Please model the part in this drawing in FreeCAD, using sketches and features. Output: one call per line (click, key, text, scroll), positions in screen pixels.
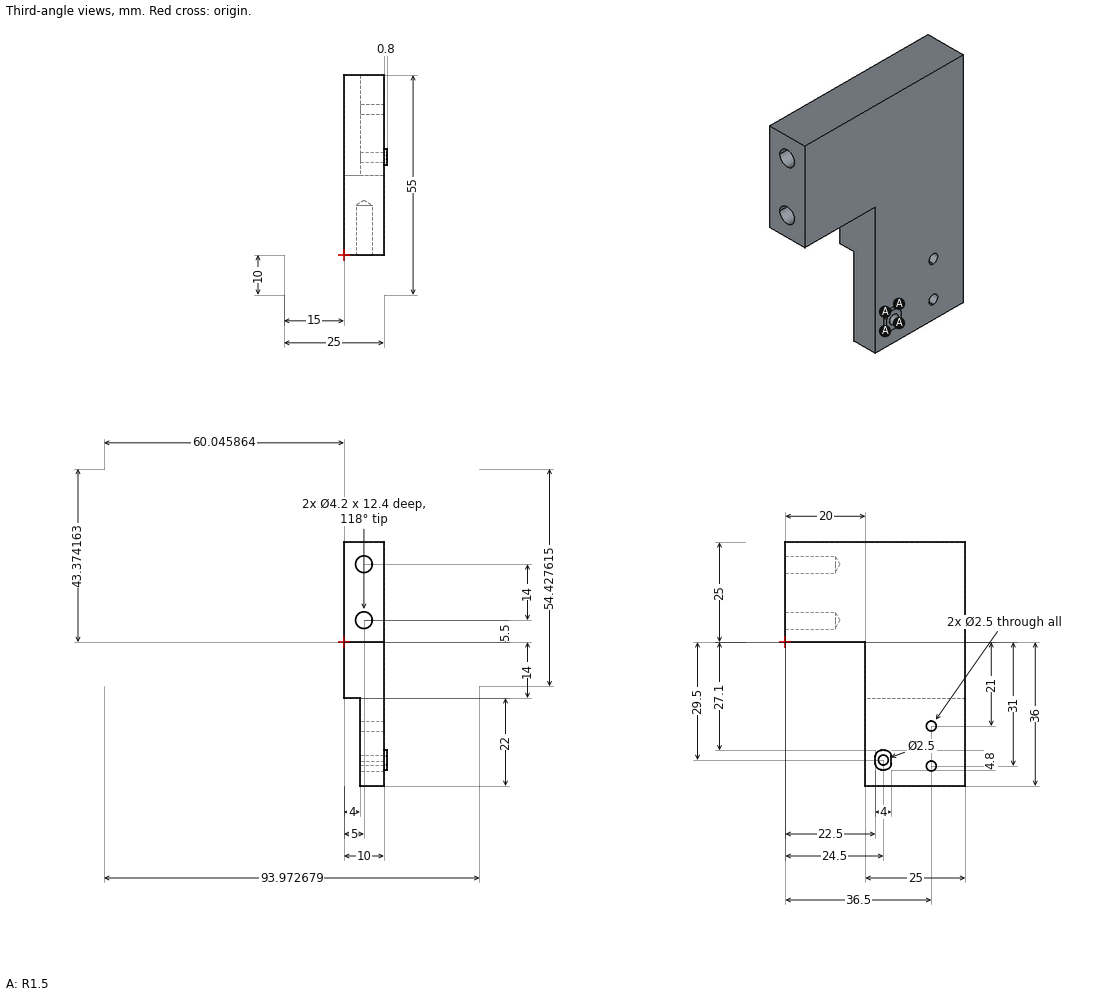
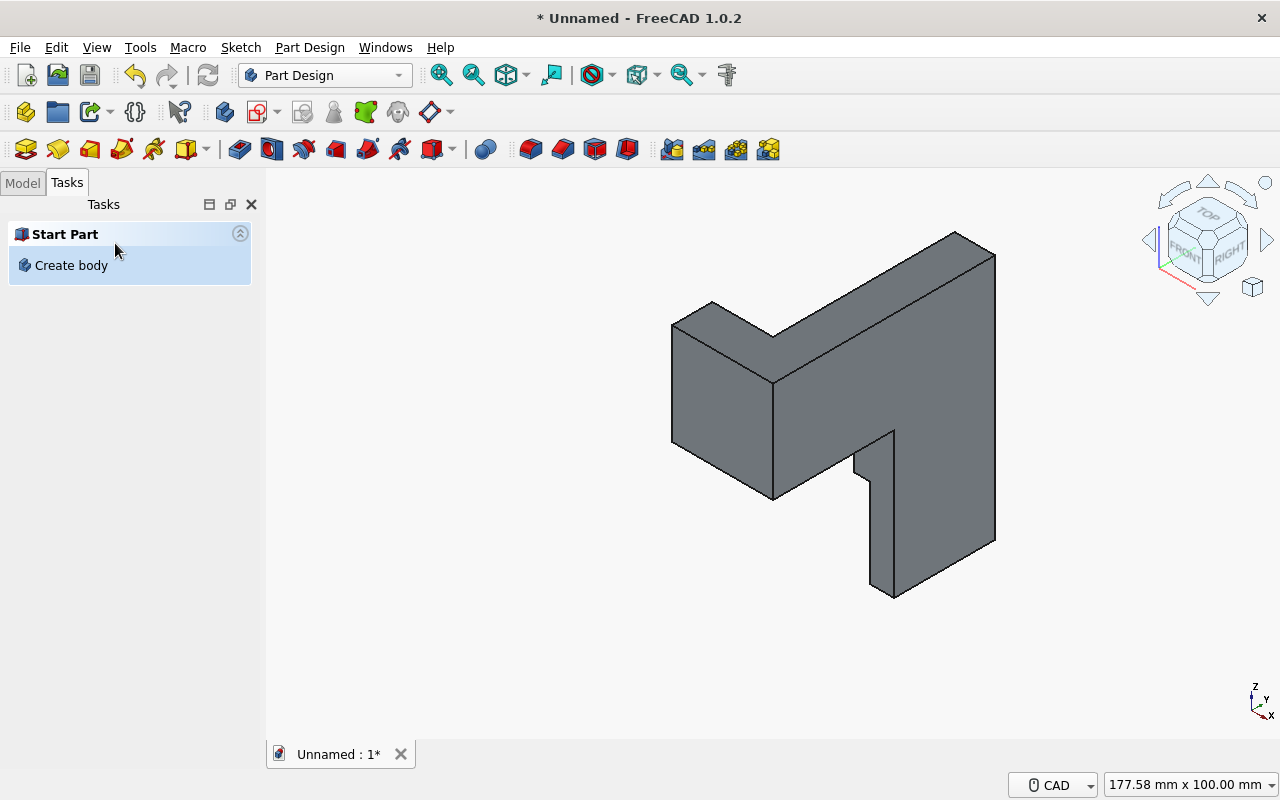
click(723, 412)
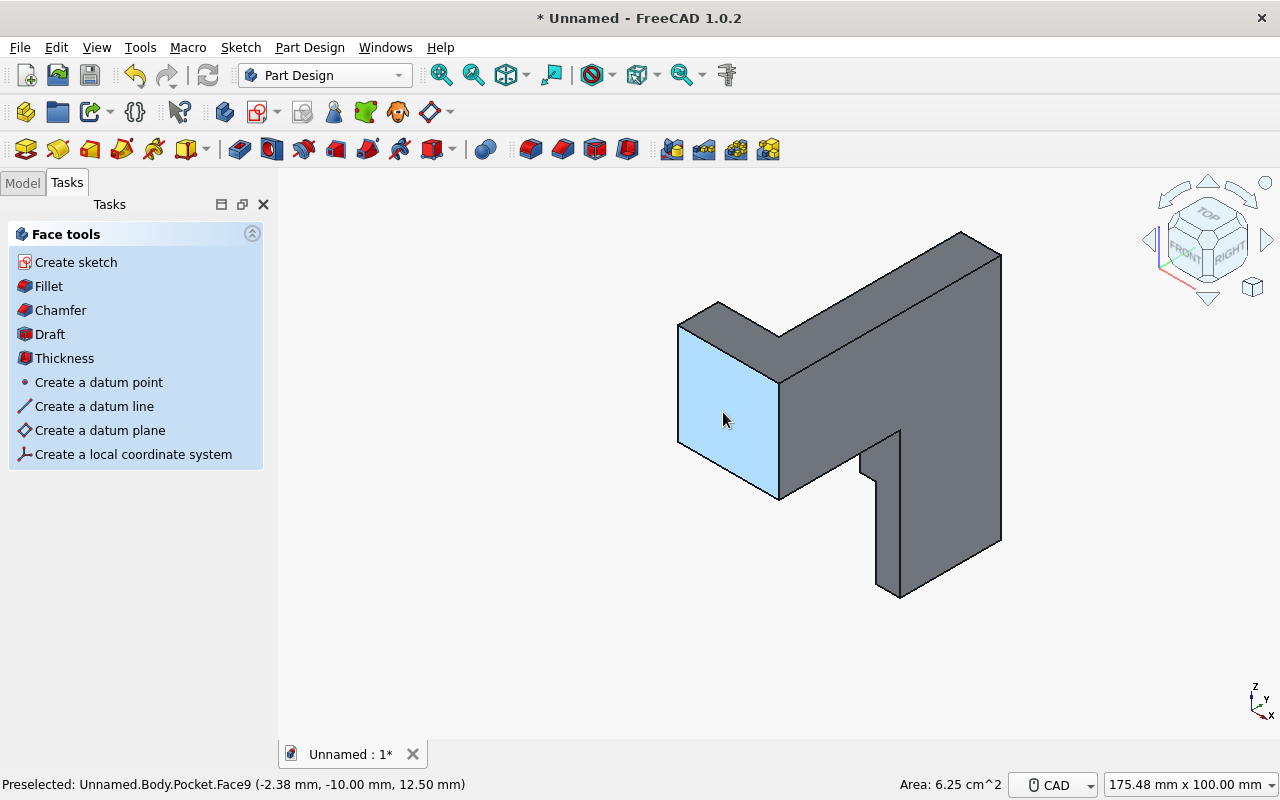
click(258, 112)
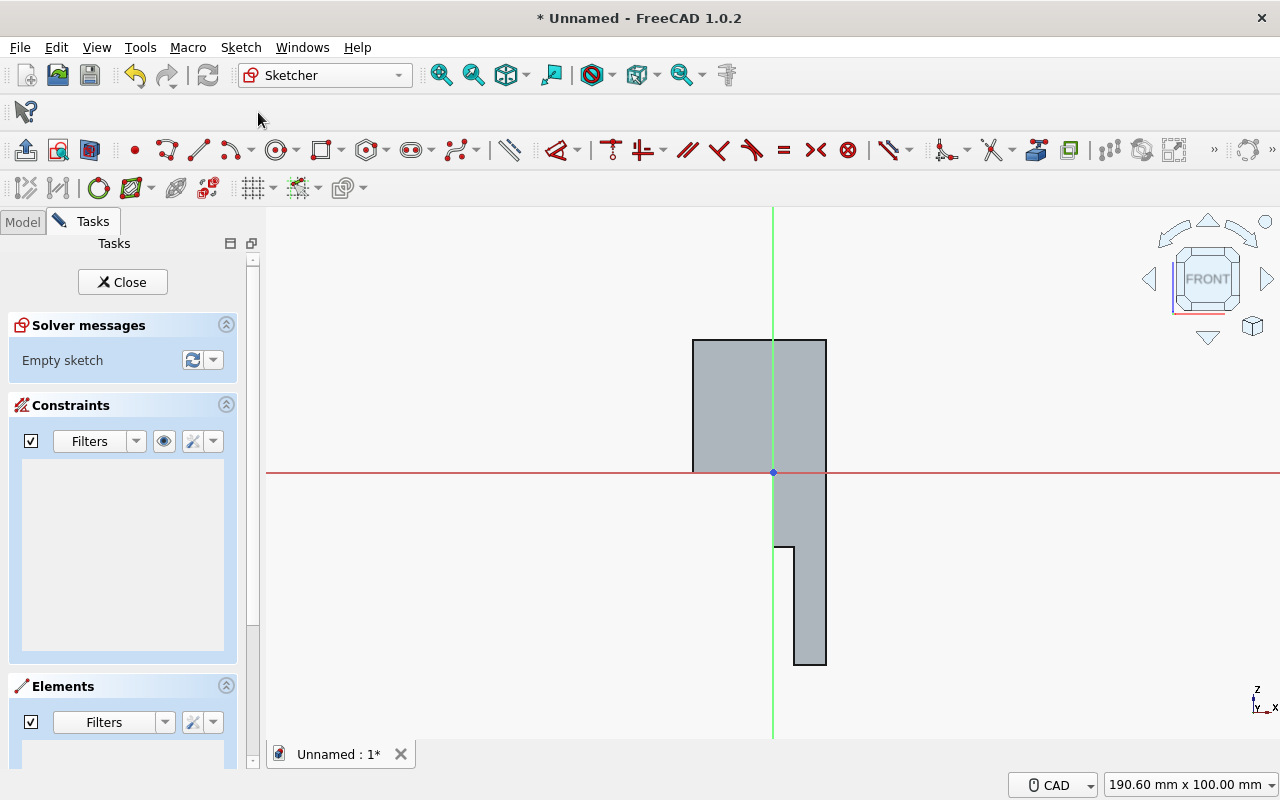
scroll(709, 711, down, 1)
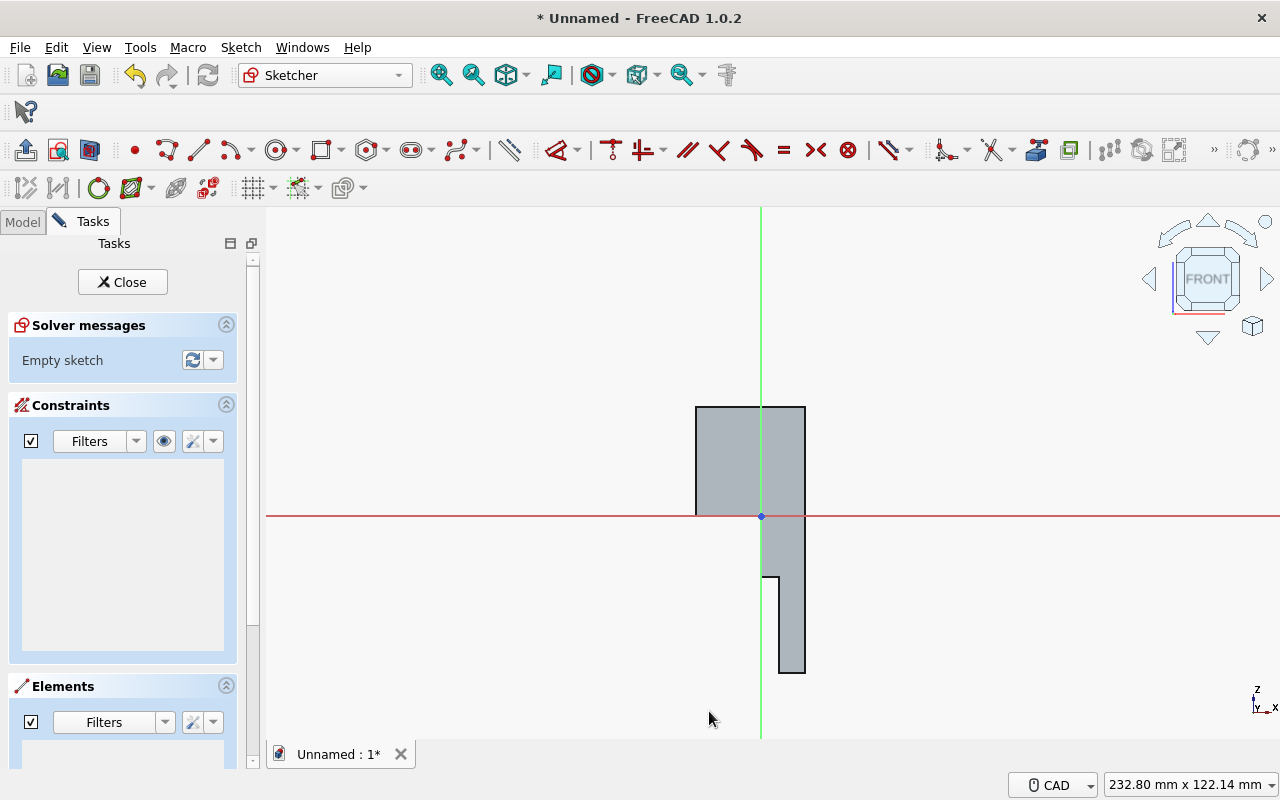
scroll(705, 391, up, 2)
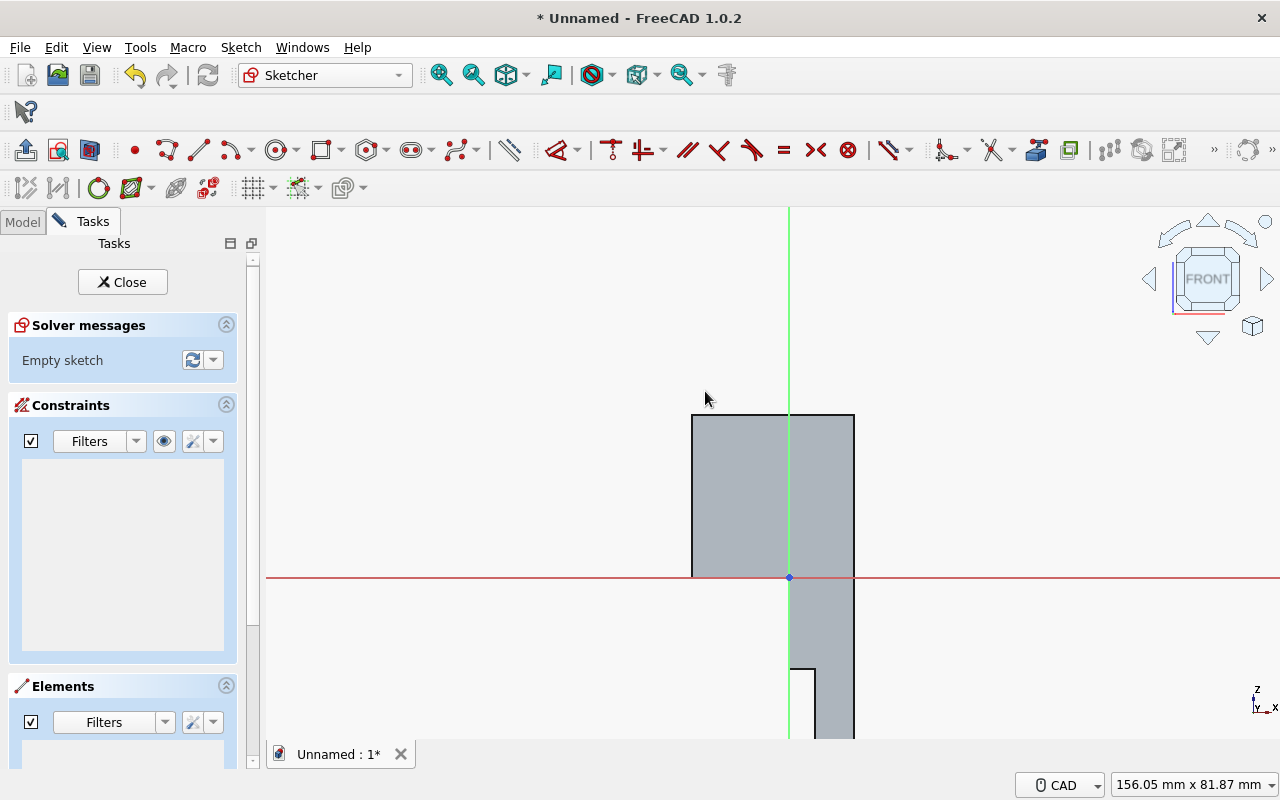
click(322, 150)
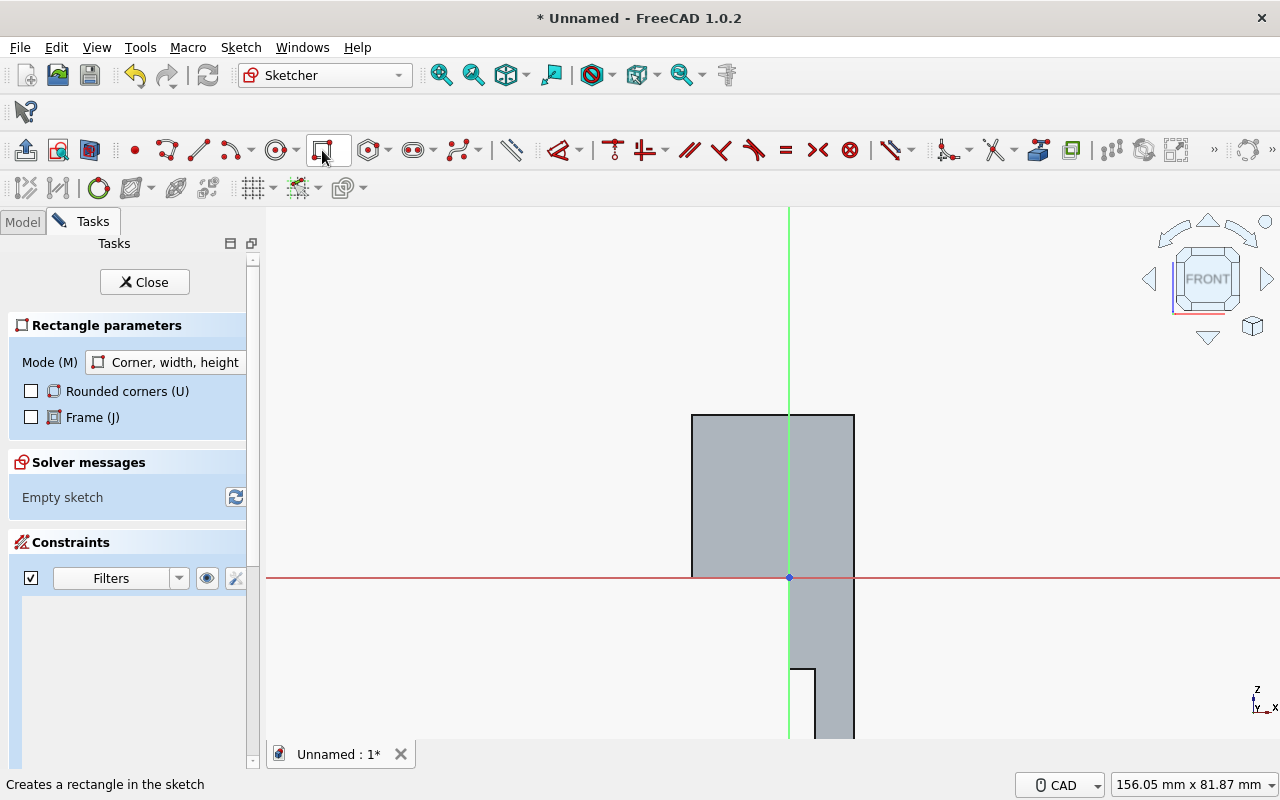
click(399, 296)
move(1009, 650)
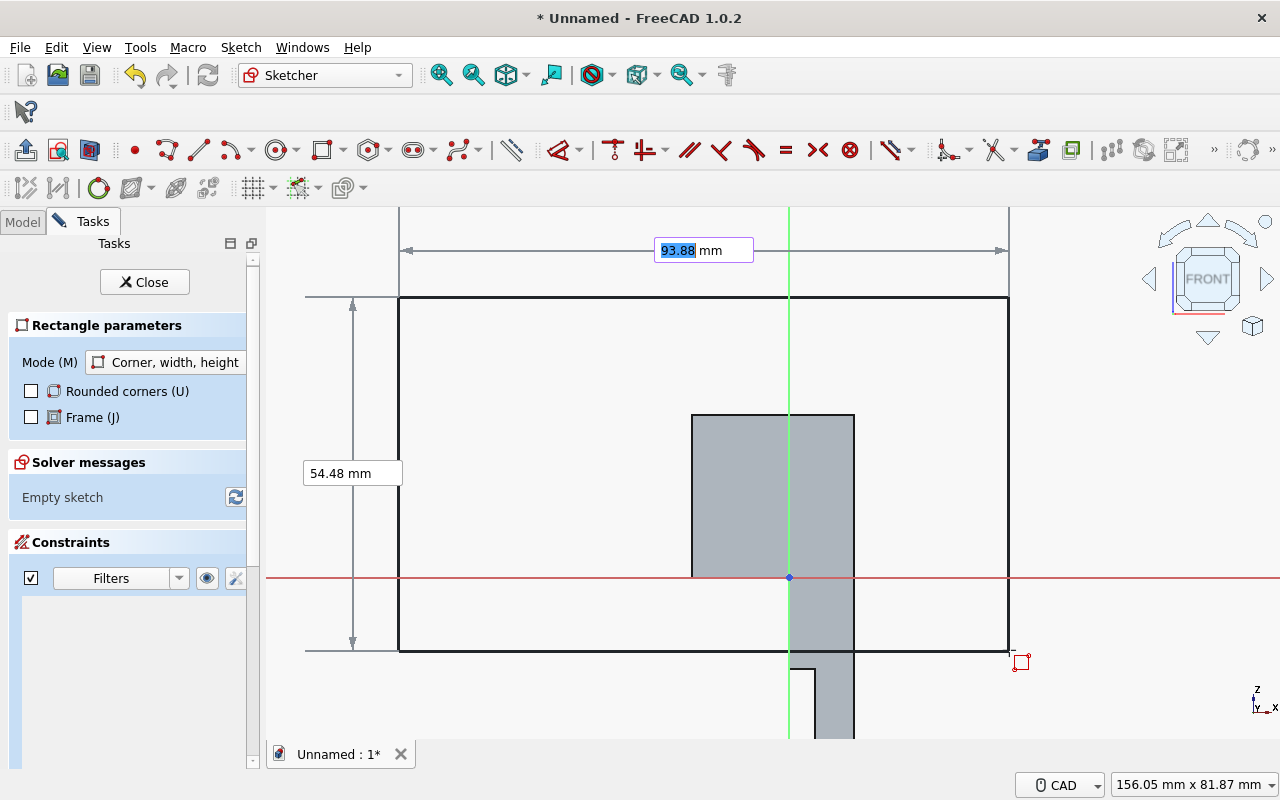
text(93.972679)
key(Tab)
text(54.427615)
key(Return)
key(Escape)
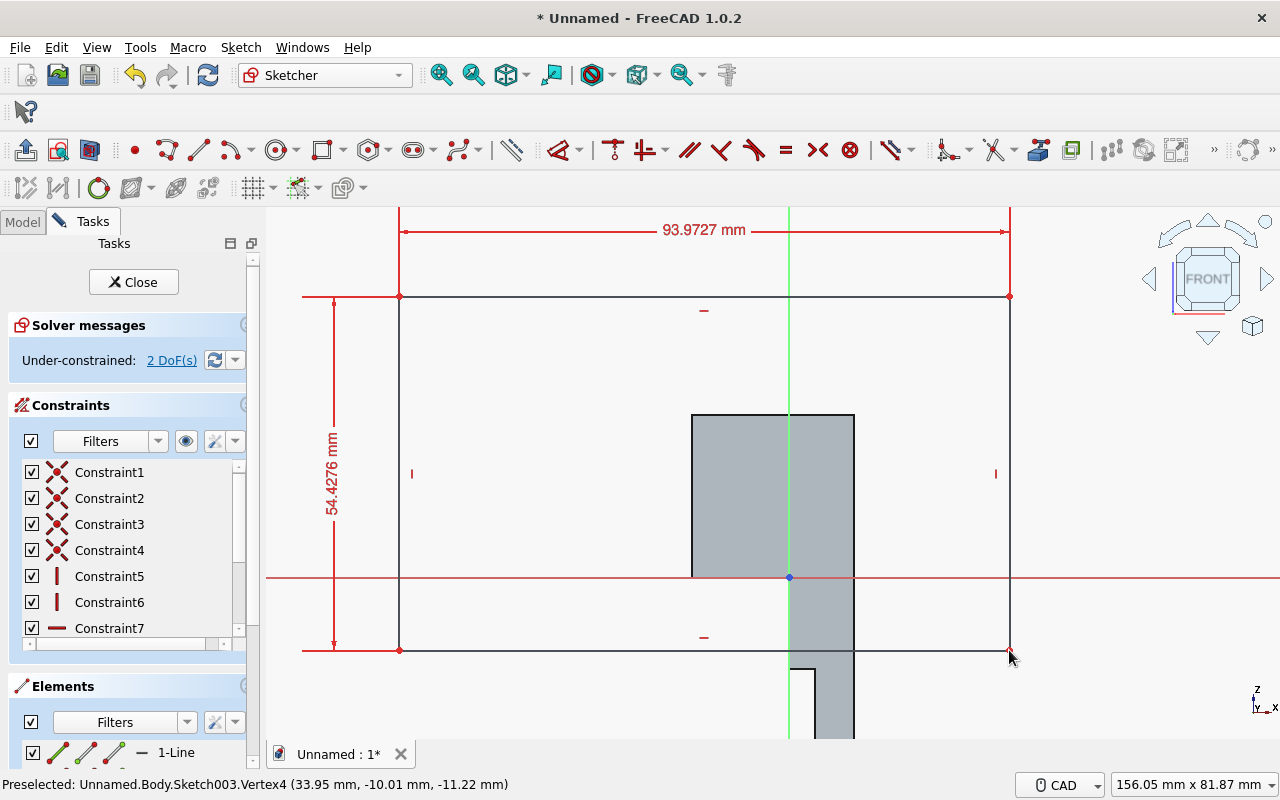
click(558, 150)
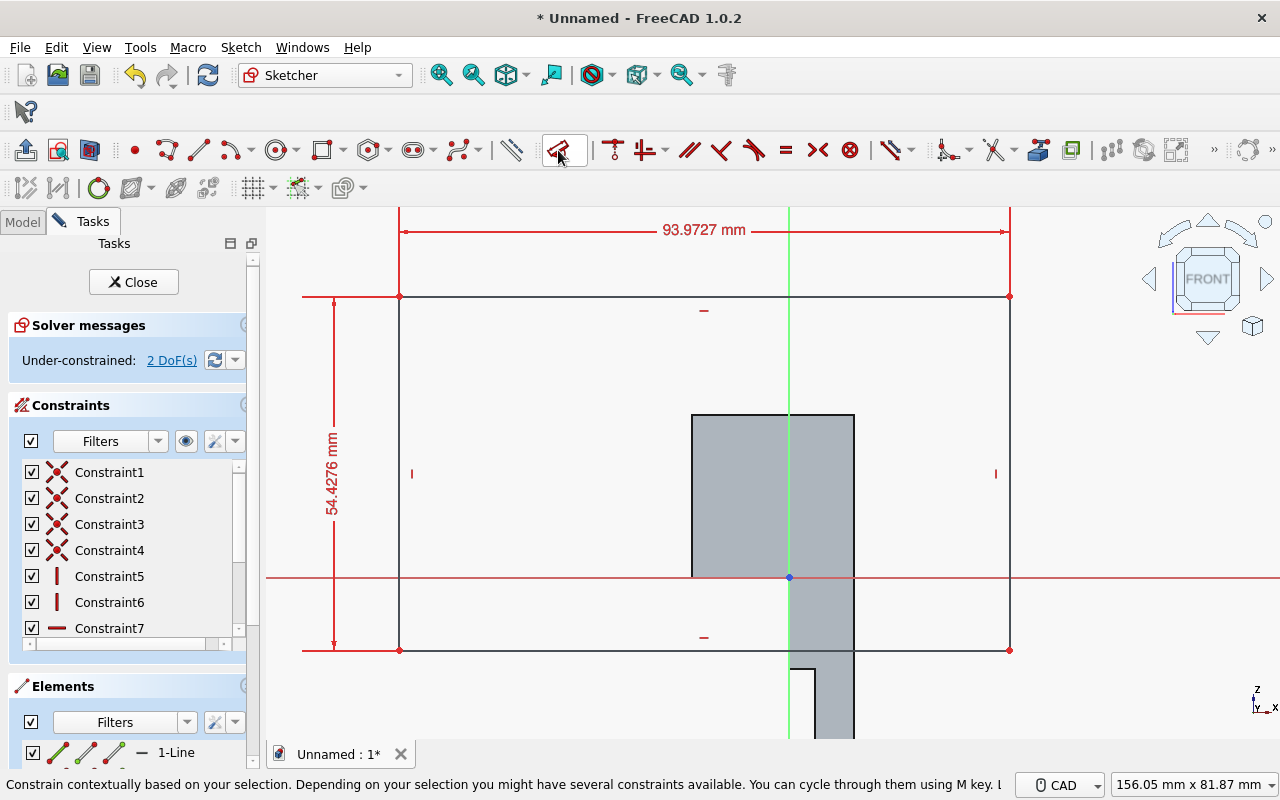
click(399, 297)
click(594, 263)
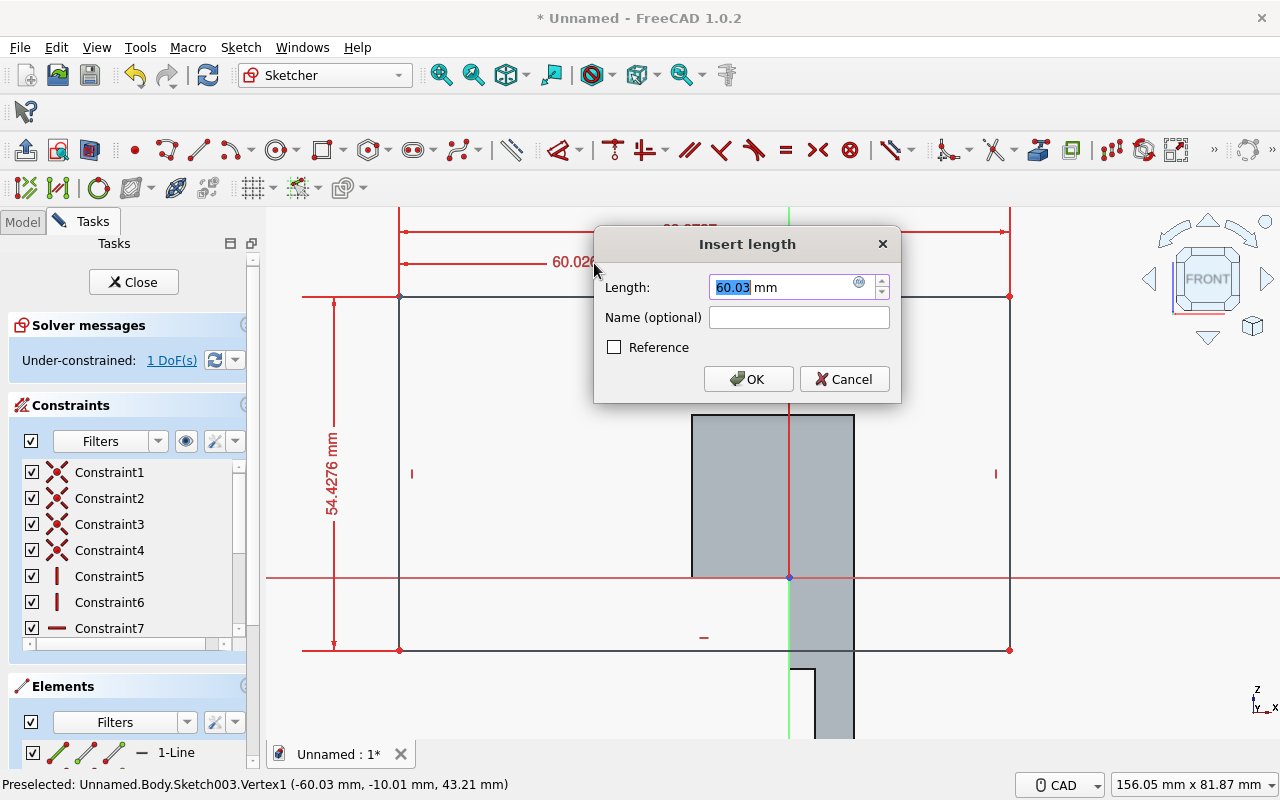
text(60.045864)
key(Return)